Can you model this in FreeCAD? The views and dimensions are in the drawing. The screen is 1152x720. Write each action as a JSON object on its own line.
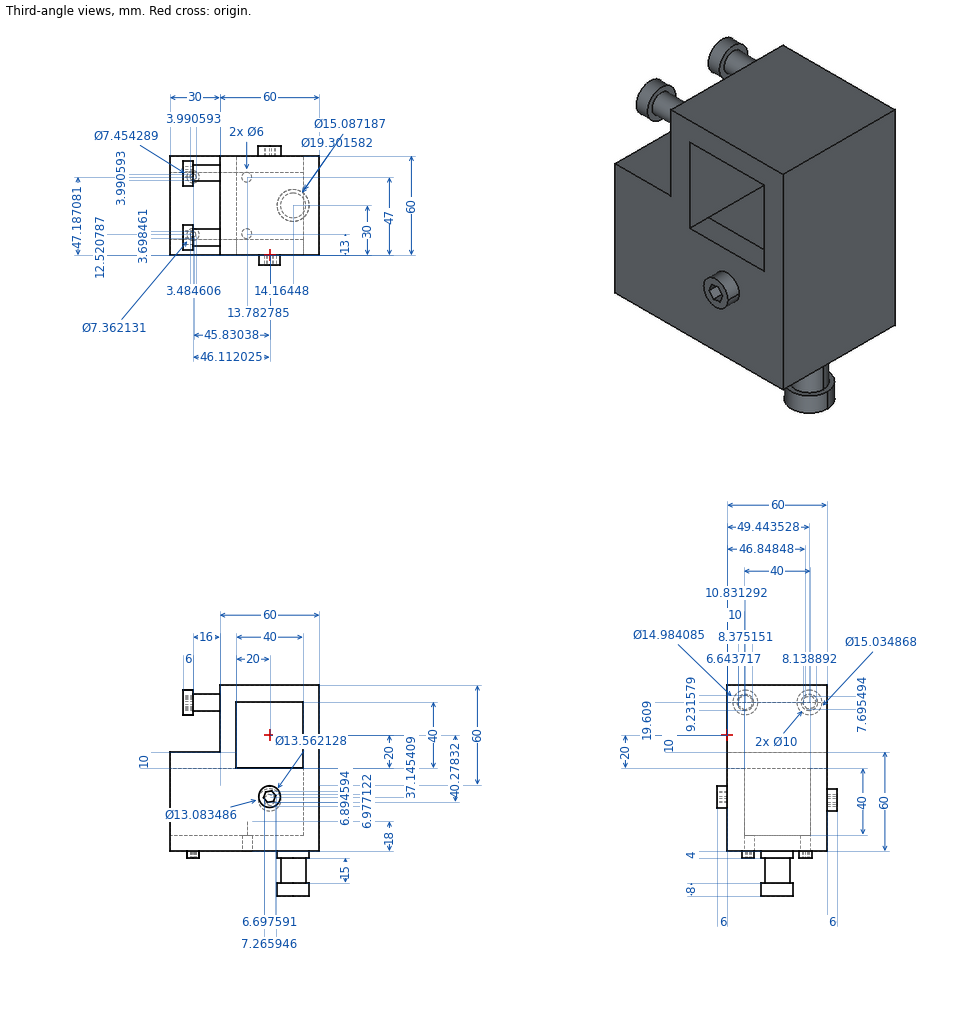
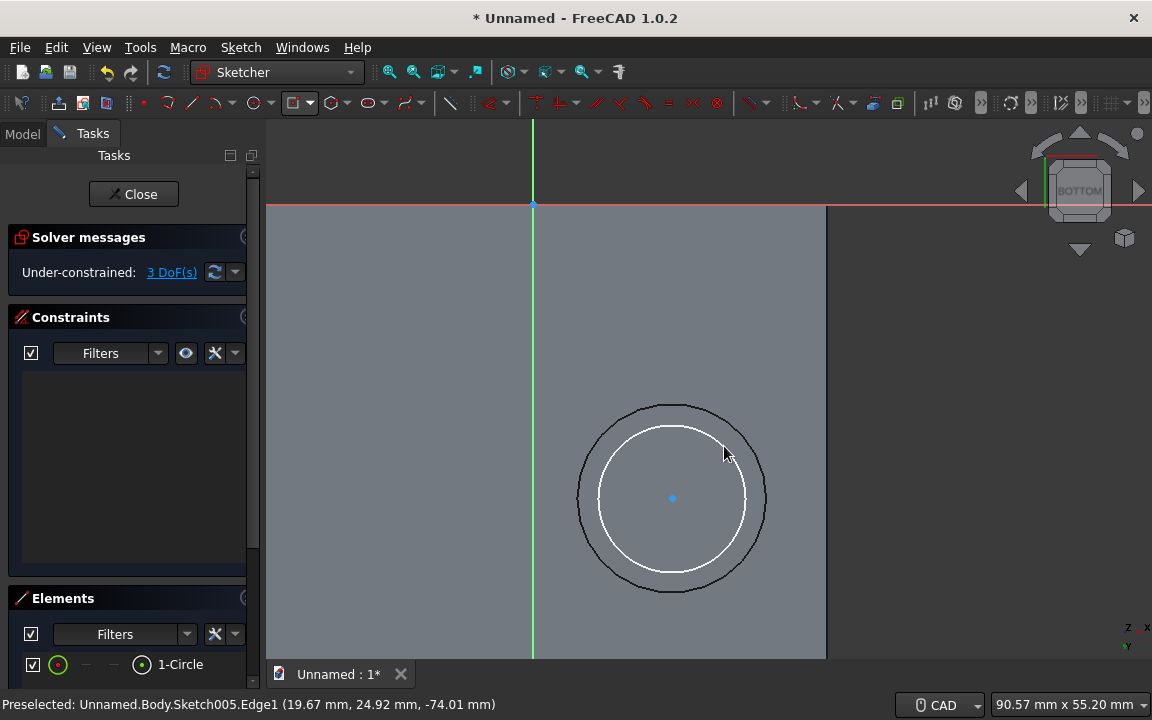
{"action": "left_click", "coordinate": [490, 104]}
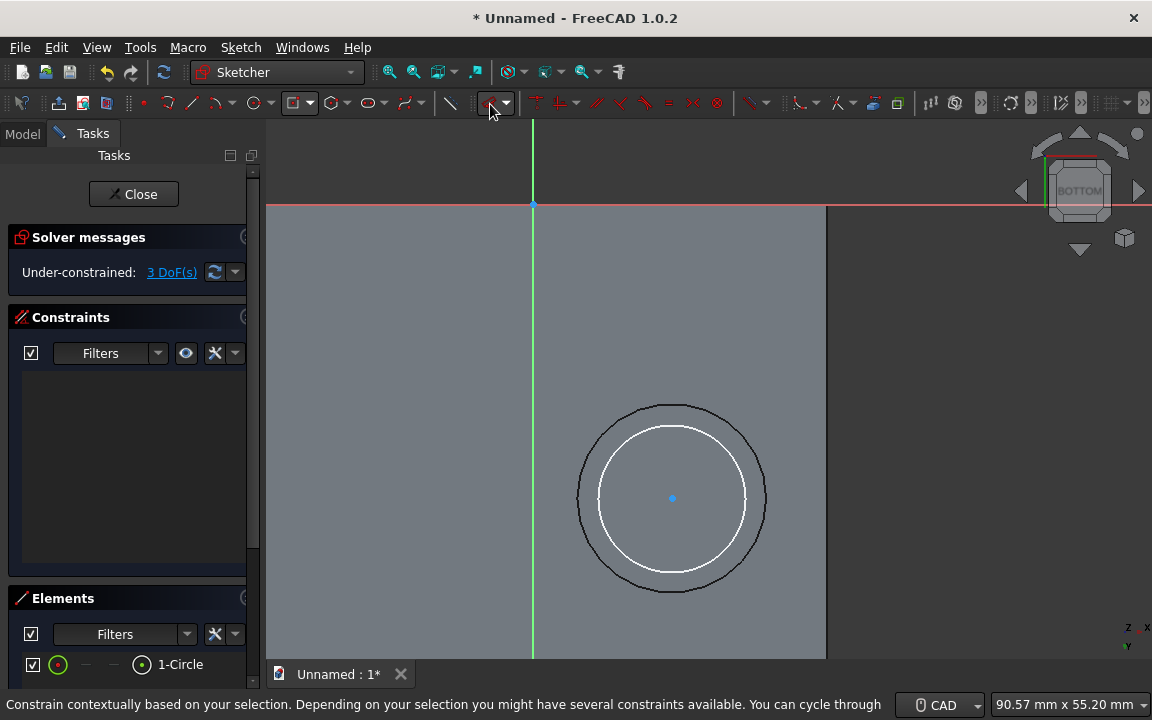
{"action": "left_click", "coordinate": [724, 447]}
{"action": "left_click", "coordinate": [747, 424]}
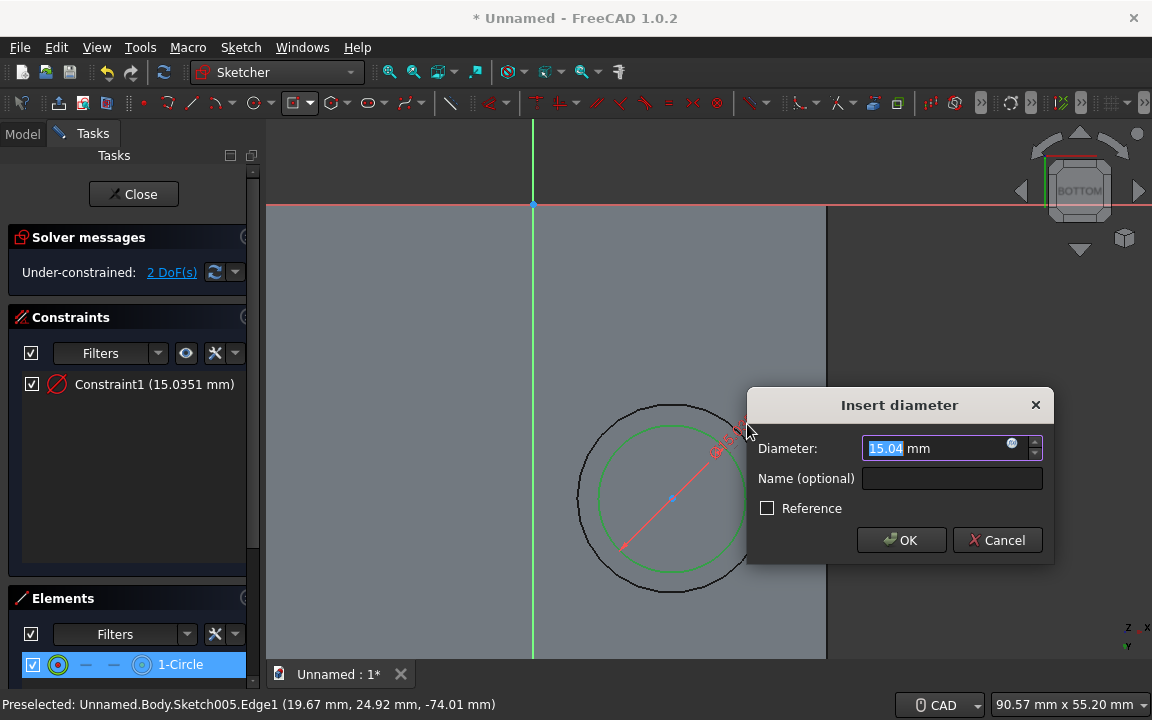
{"action": "type", "text": "15.087187"}
{"action": "key", "text": "Return"}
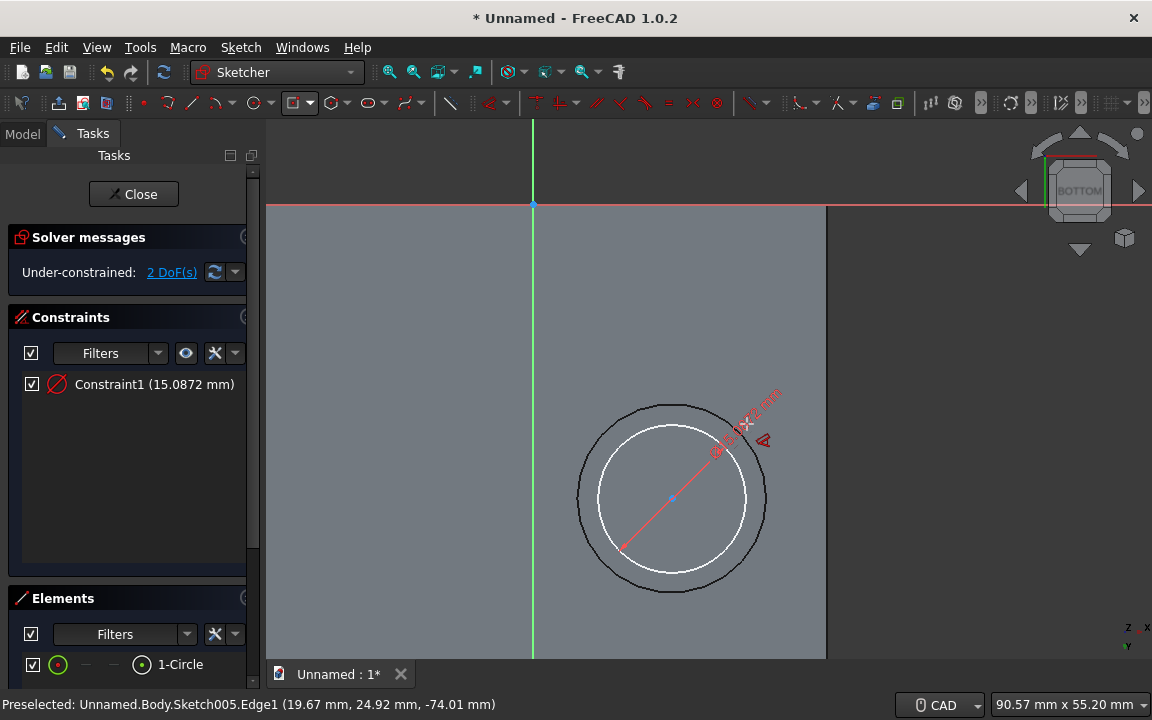
{"action": "left_click", "coordinate": [672, 499]}
{"action": "left_click", "coordinate": [499, 352]}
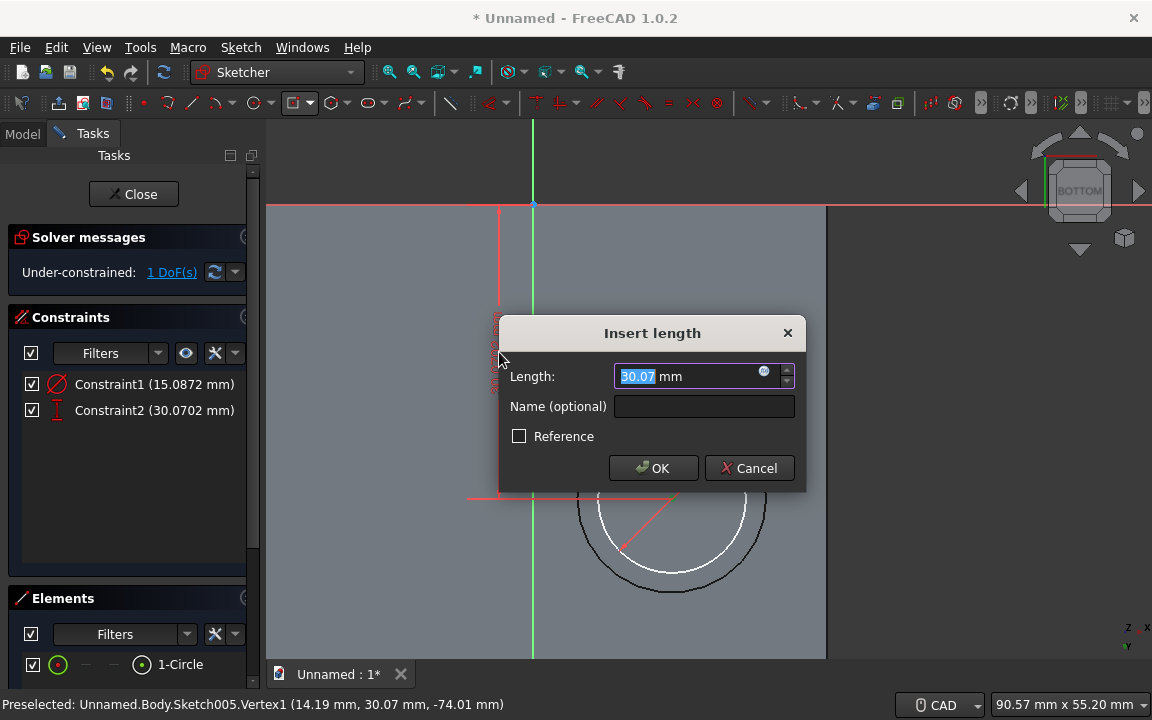
{"action": "type", "text": "30"}
{"action": "key", "text": "Return"}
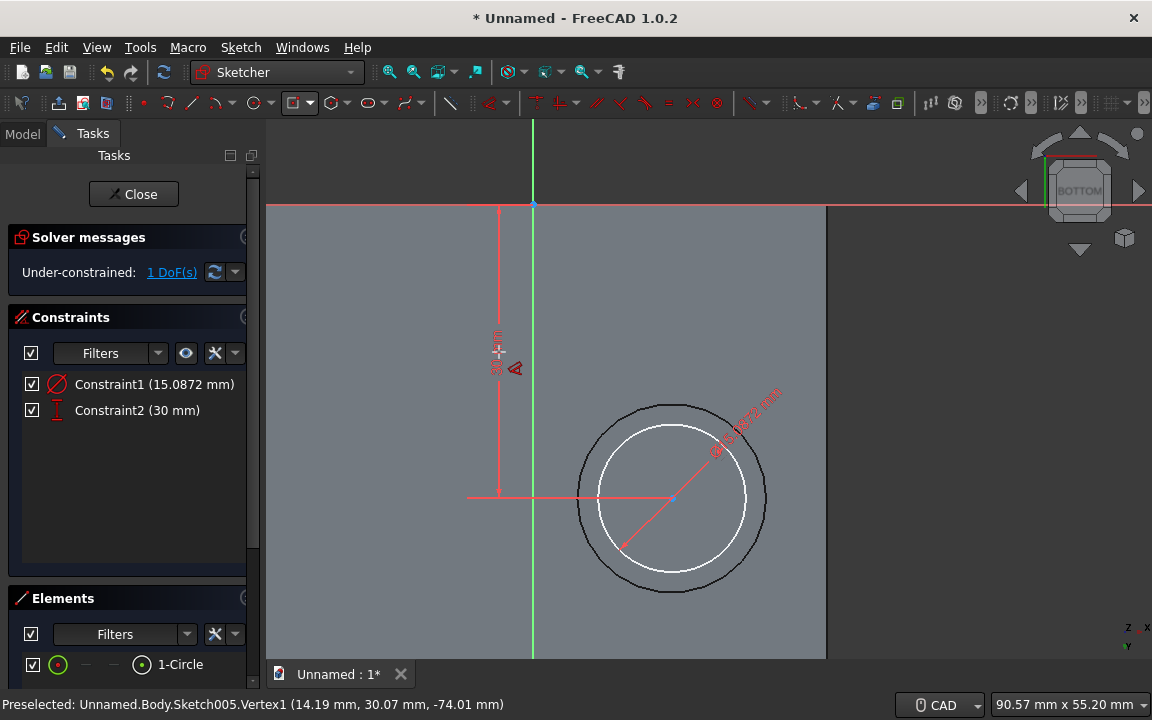
{"action": "left_click", "coordinate": [672, 498]}
{"action": "left_click", "coordinate": [603, 171]}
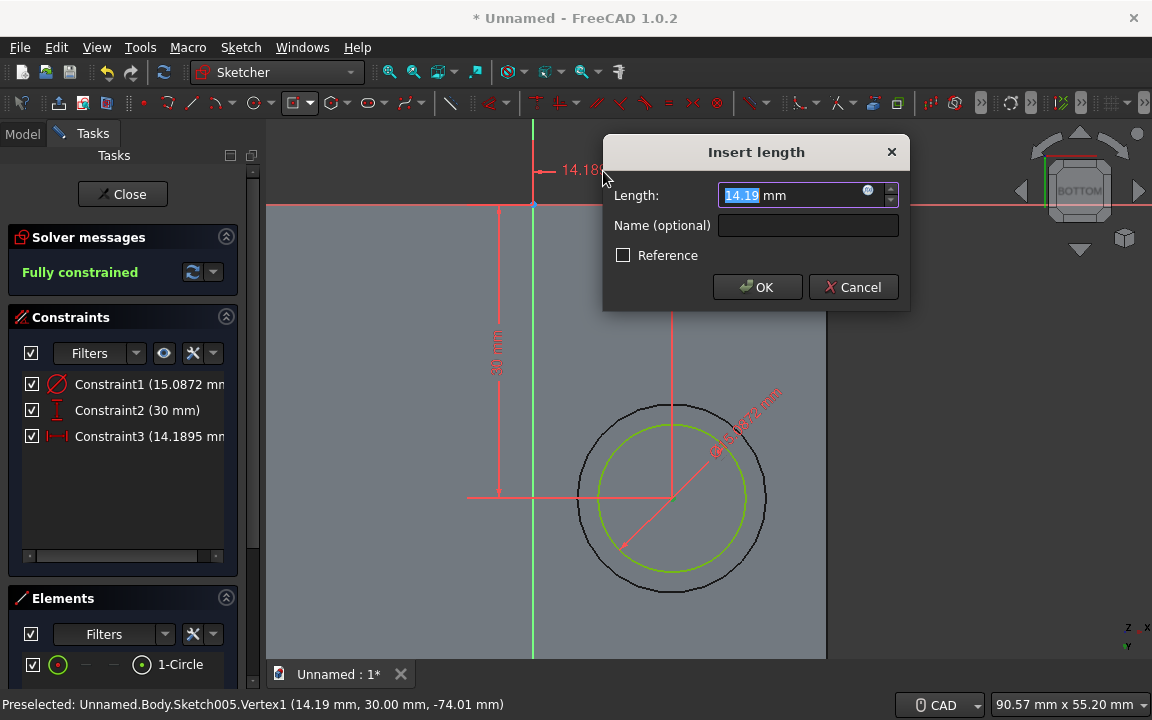
{"action": "type", "text": "14.16448"}
{"action": "key", "text": "Return"}
{"action": "key", "text": "Escape"}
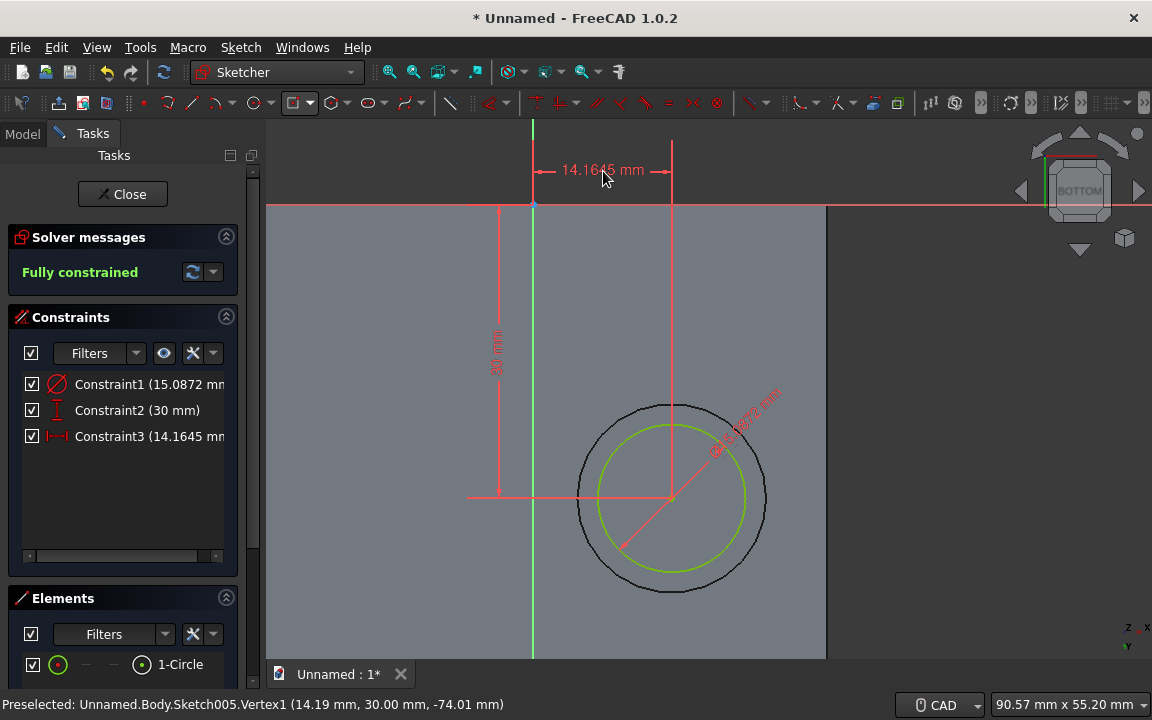
{"action": "left_click", "coordinate": [123, 194]}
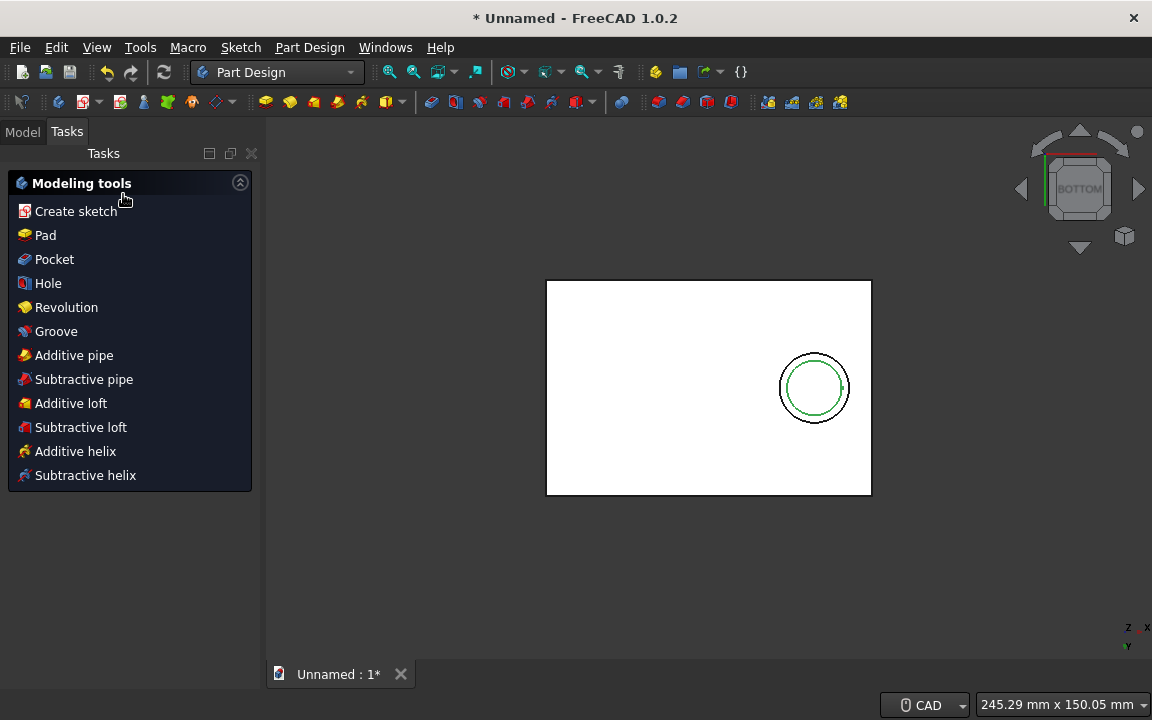
{"action": "left_click", "coordinate": [266, 102]}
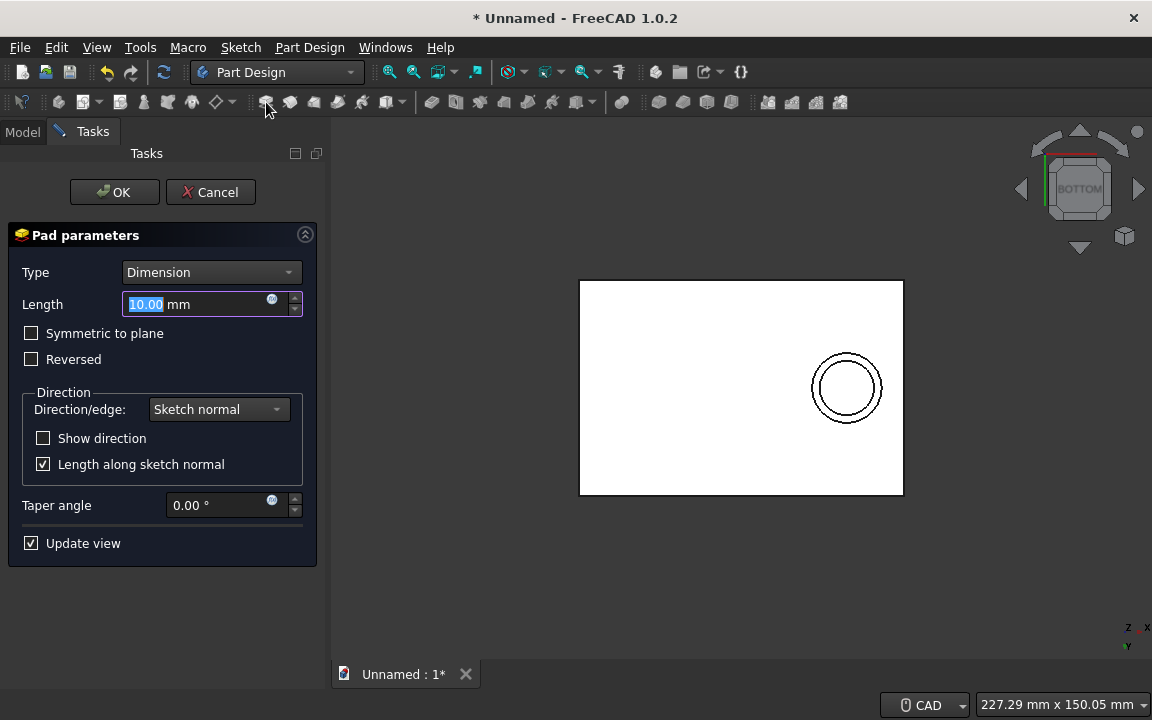
{"action": "type", "text": "15"}
{"action": "key", "text": "Tab"}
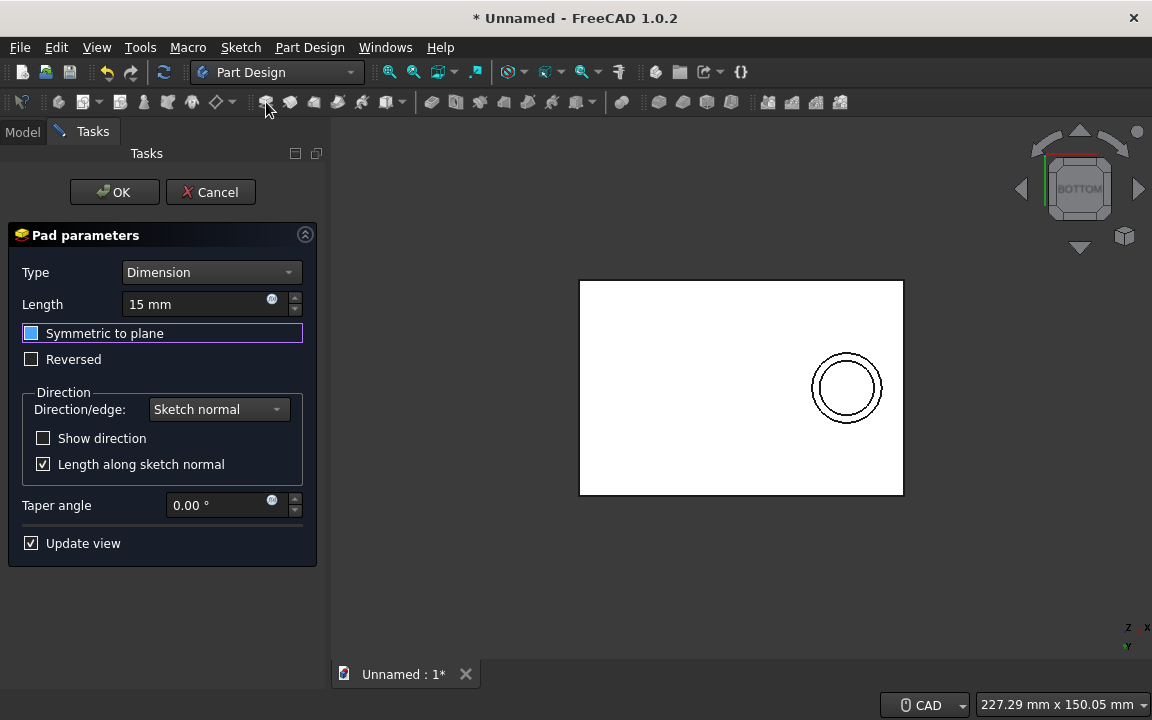
{"action": "left_click", "coordinate": [115, 192]}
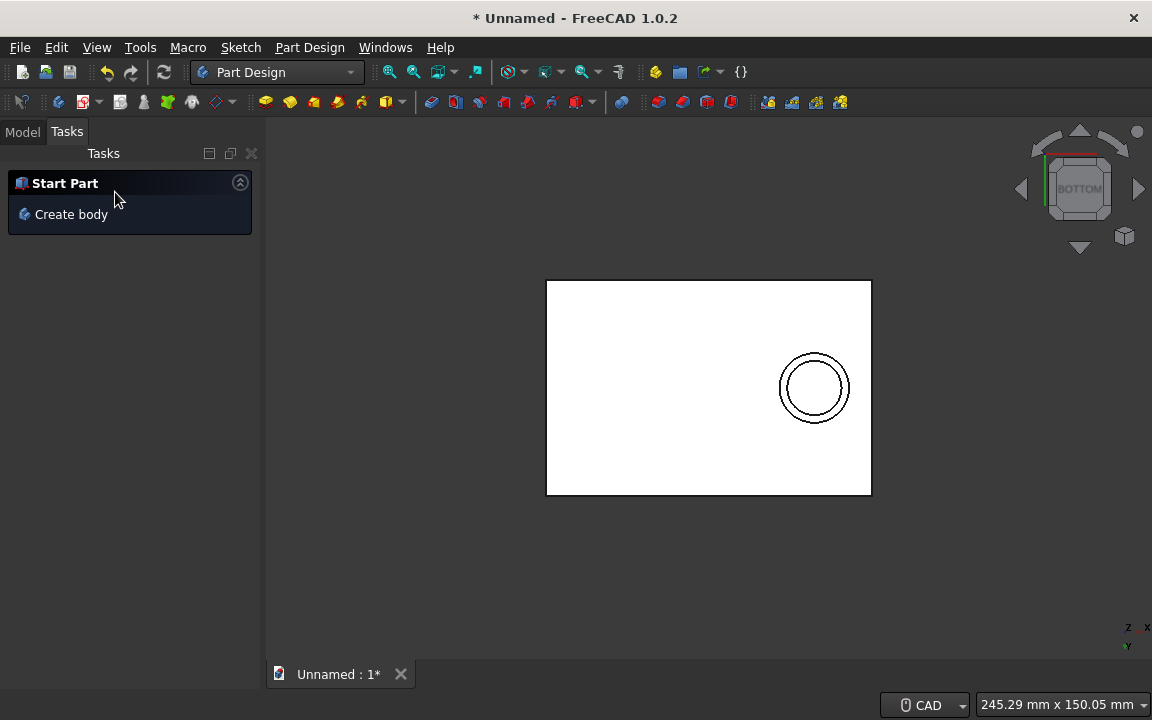
{"action": "left_click", "coordinate": [390, 72]}